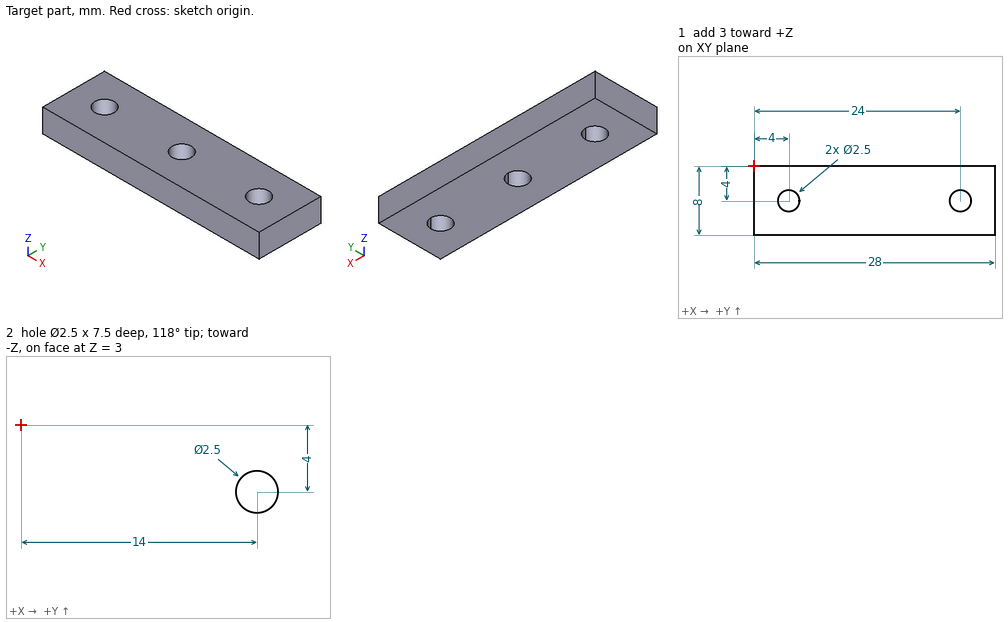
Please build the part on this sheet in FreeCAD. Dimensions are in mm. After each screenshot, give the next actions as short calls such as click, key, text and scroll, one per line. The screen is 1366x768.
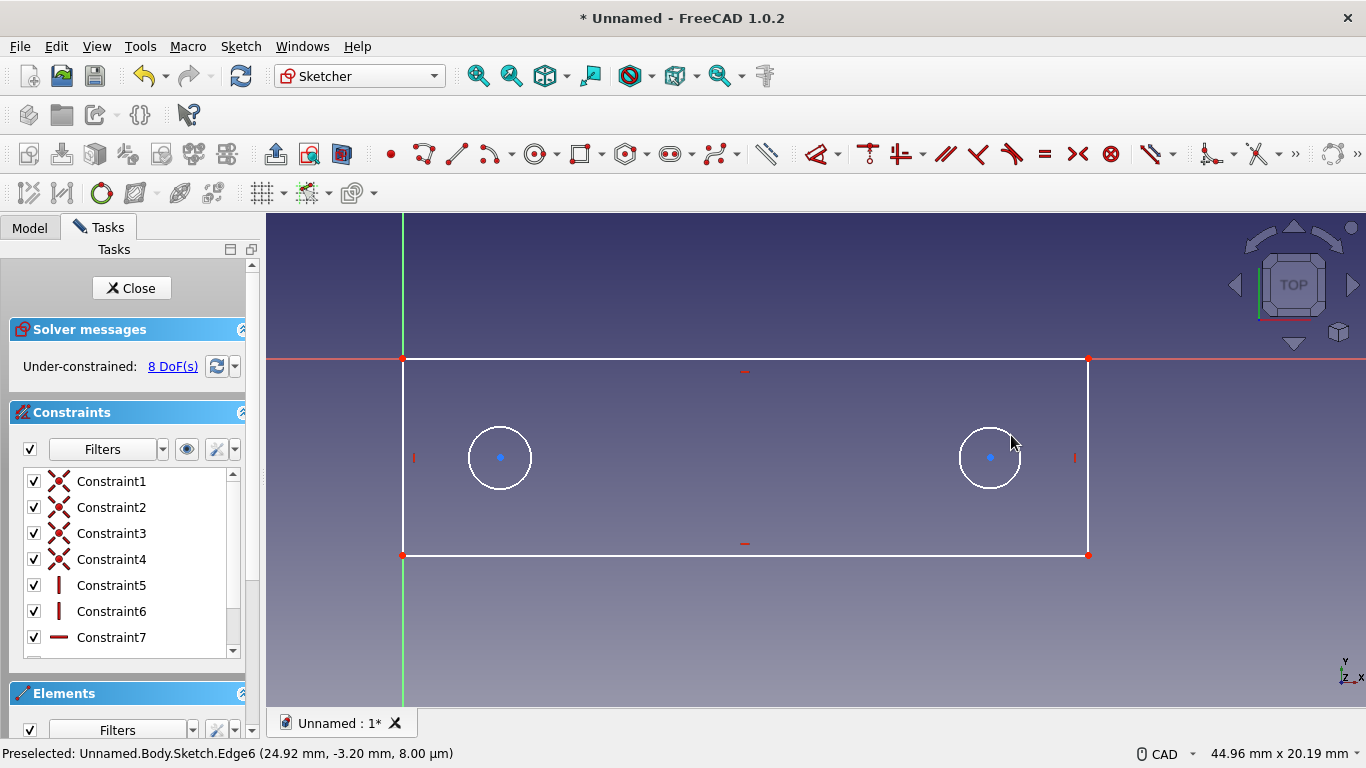
click(522, 436)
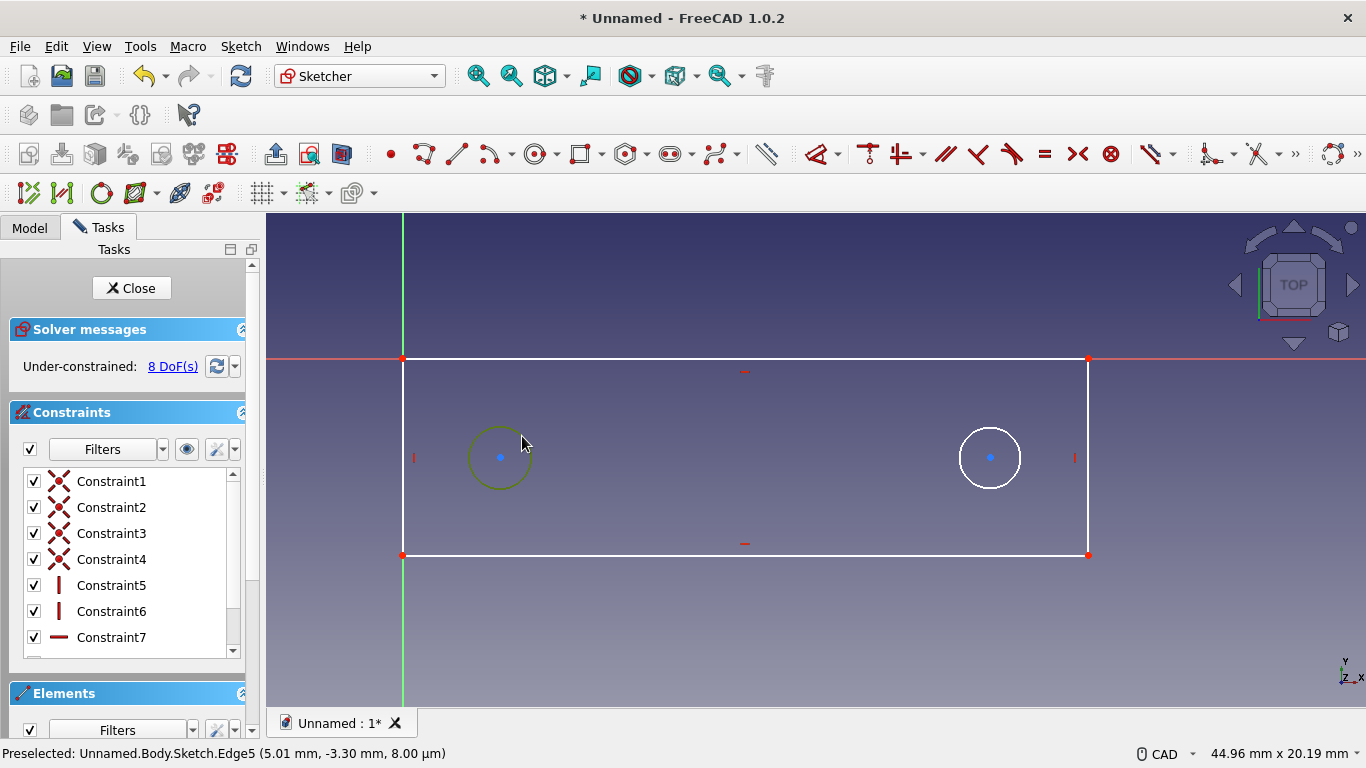
click(1011, 436)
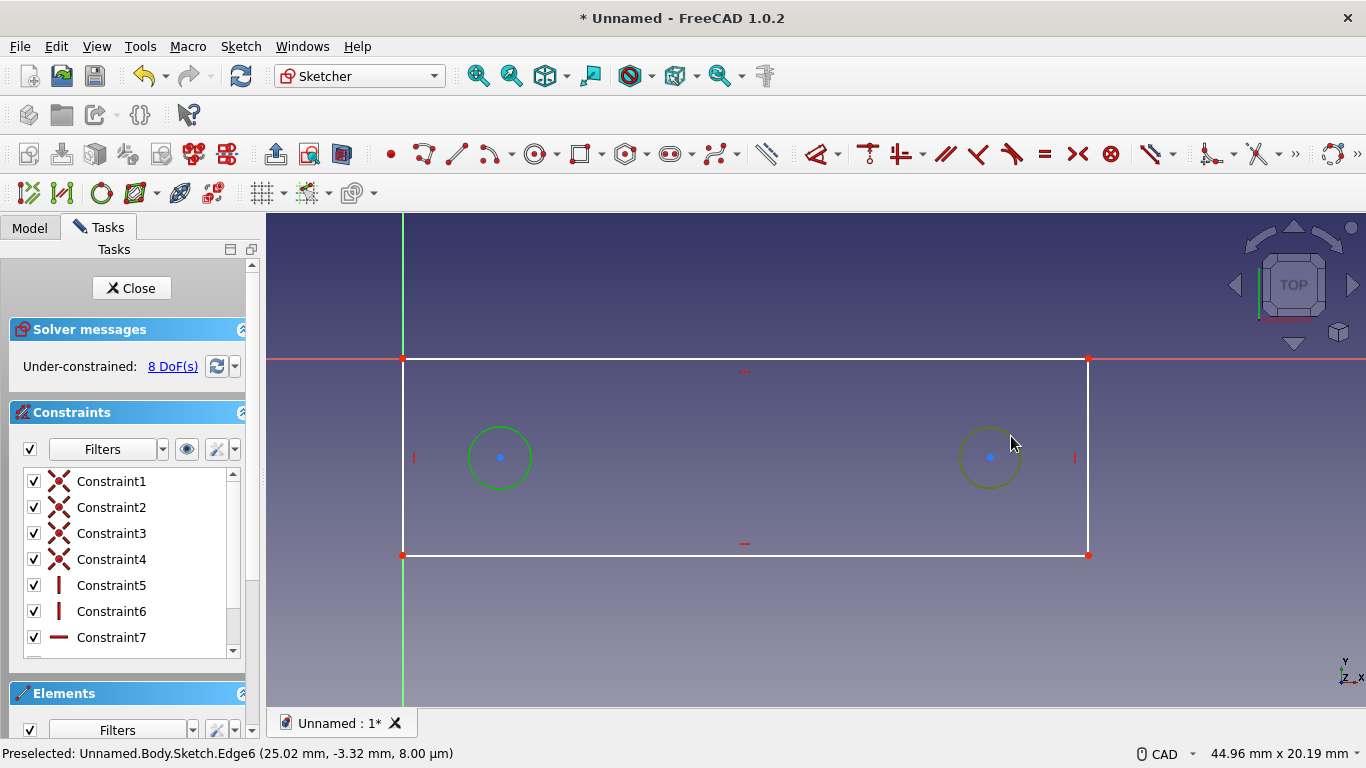
click(1045, 154)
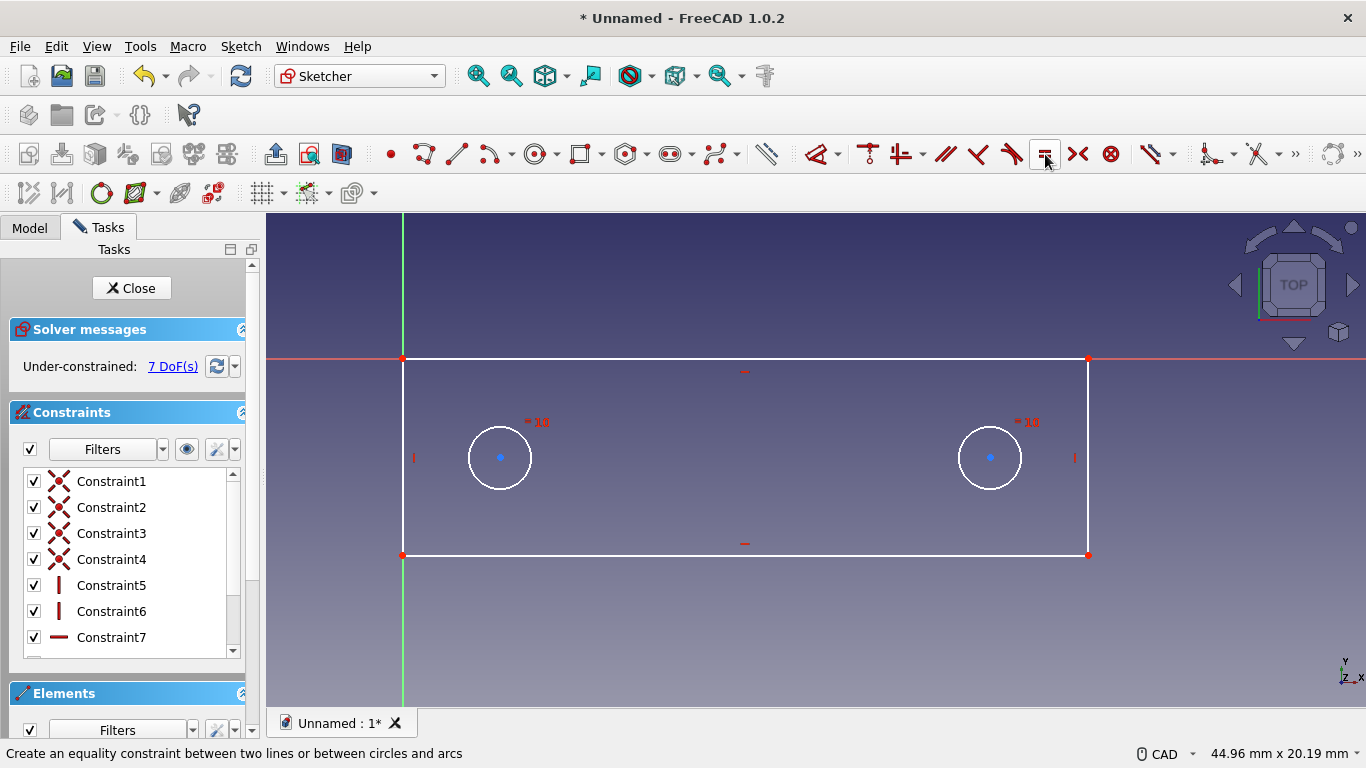
click(500, 458)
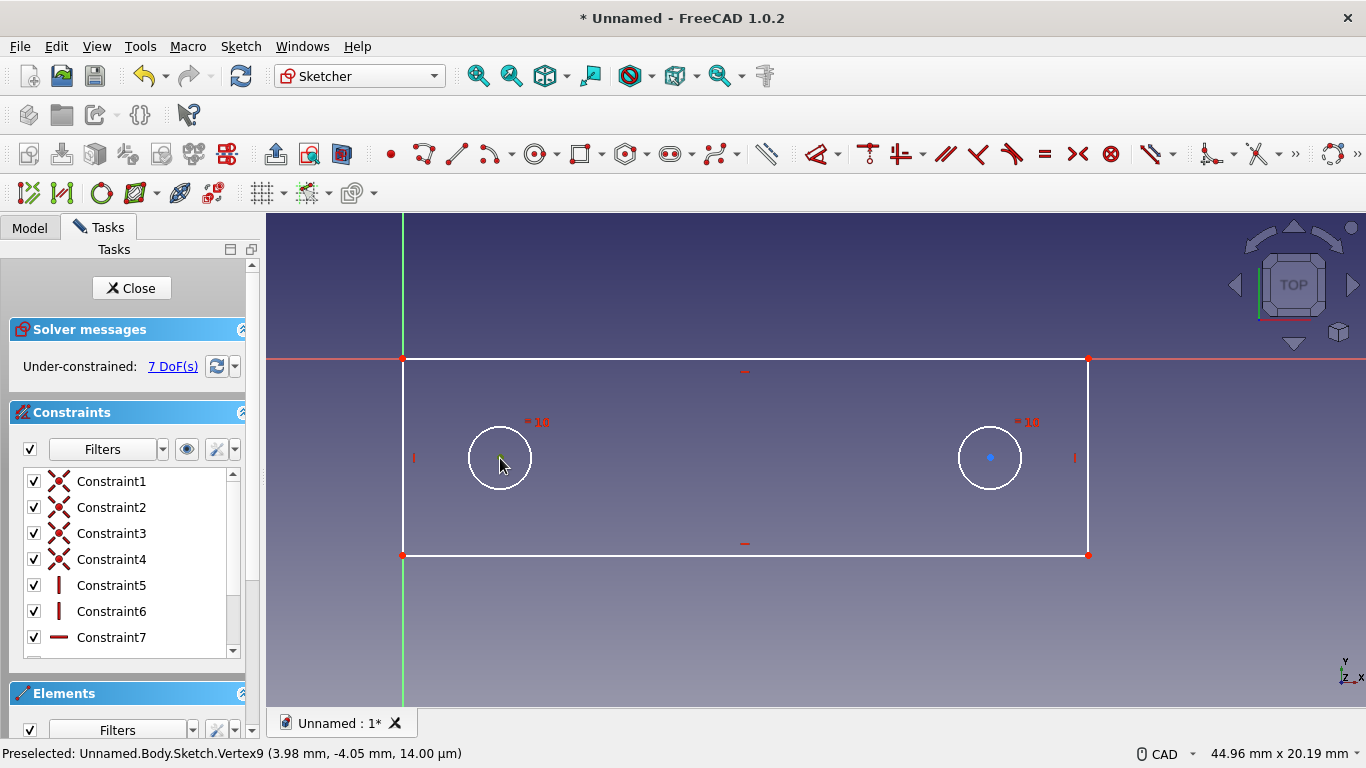
click(990, 458)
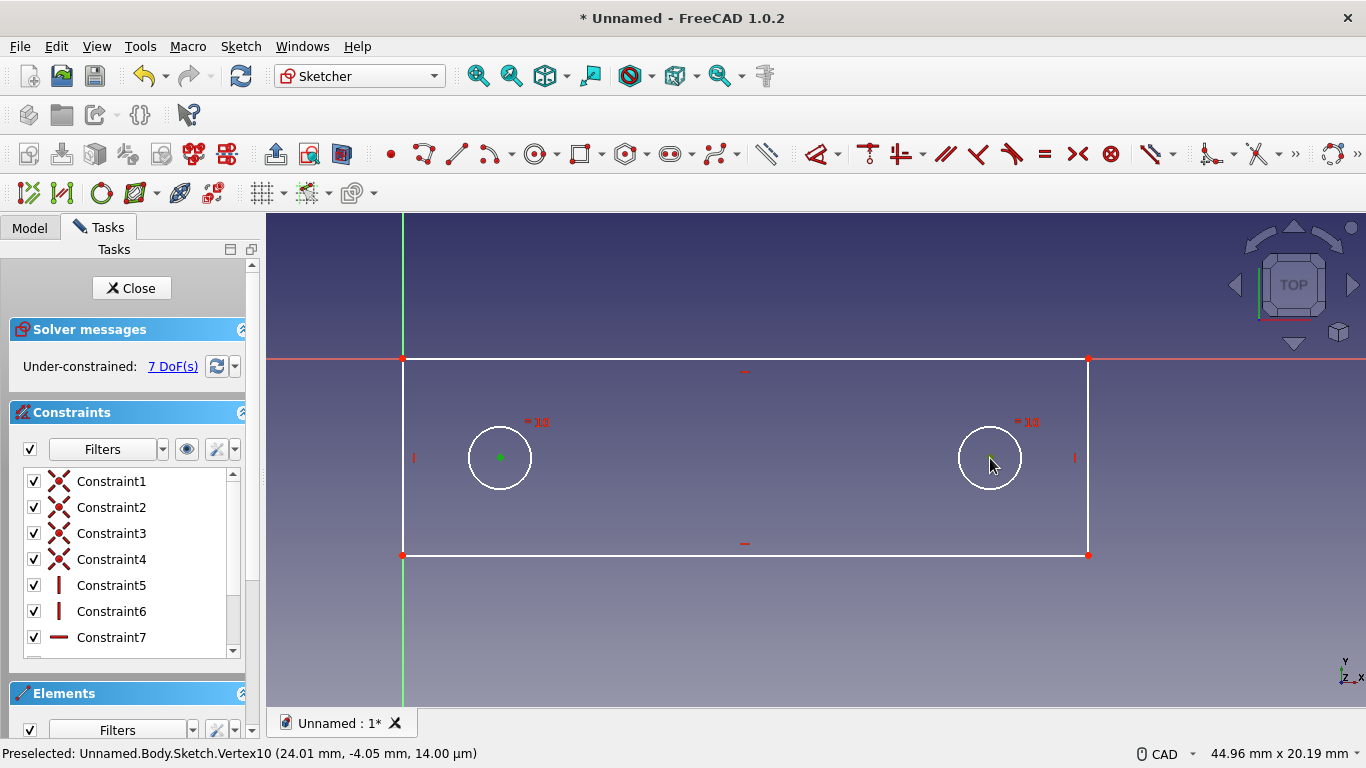
key(h)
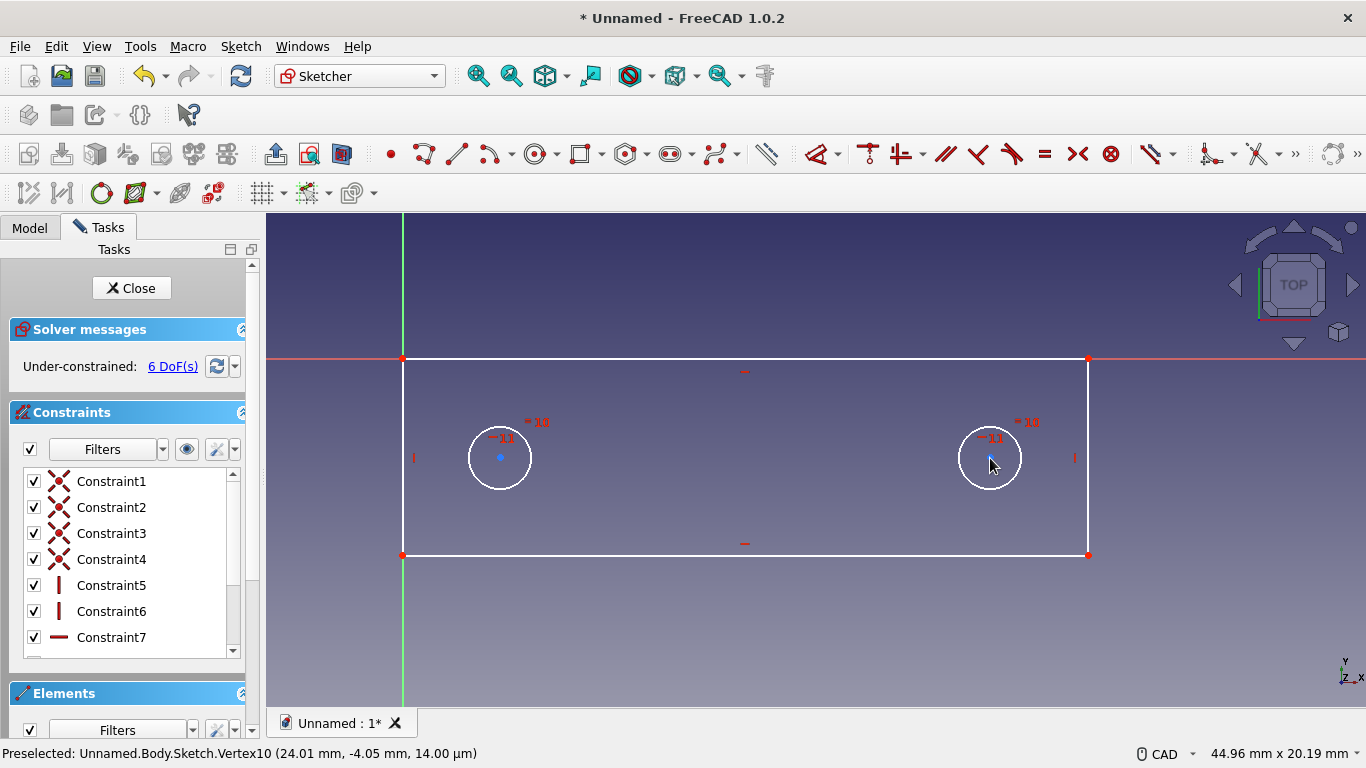
click(816, 154)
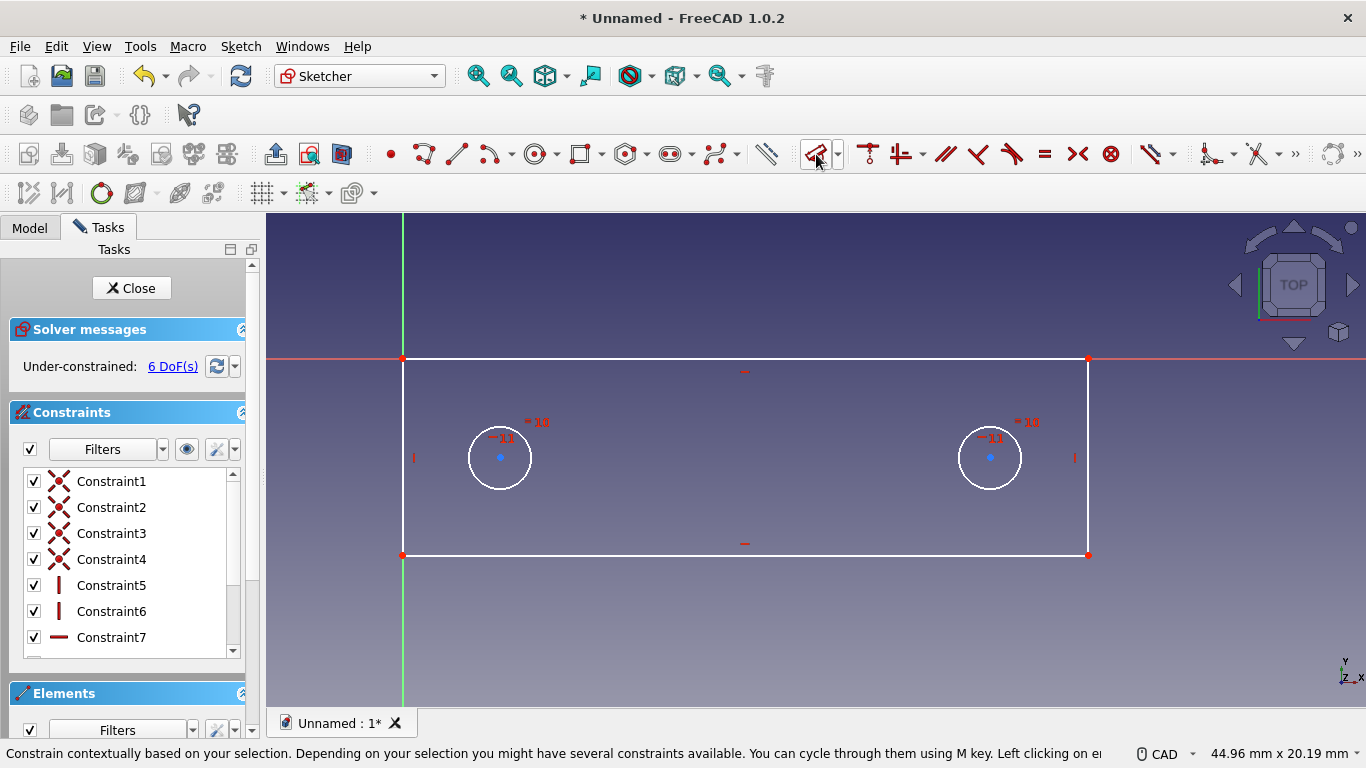
click(522, 436)
click(545, 413)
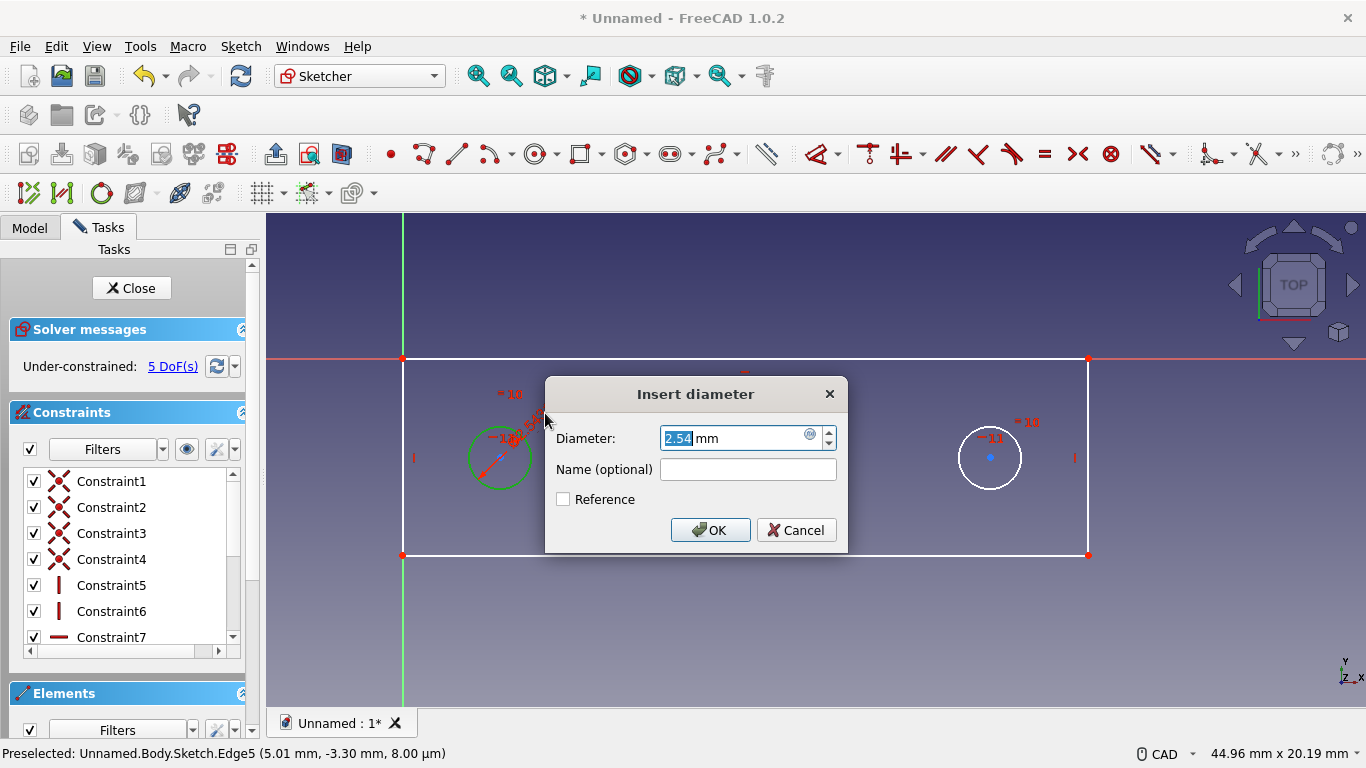
text(2.5)
key(Return)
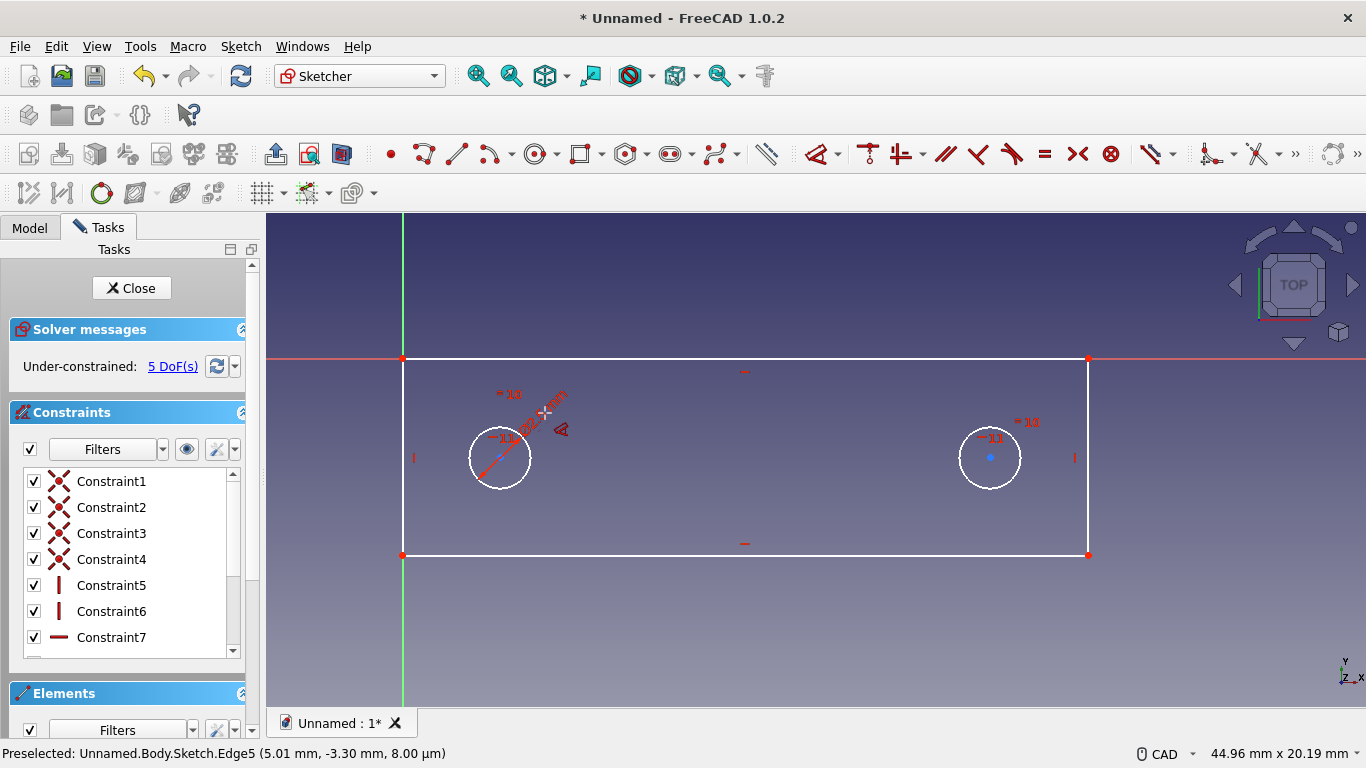
click(403, 418)
click(369, 457)